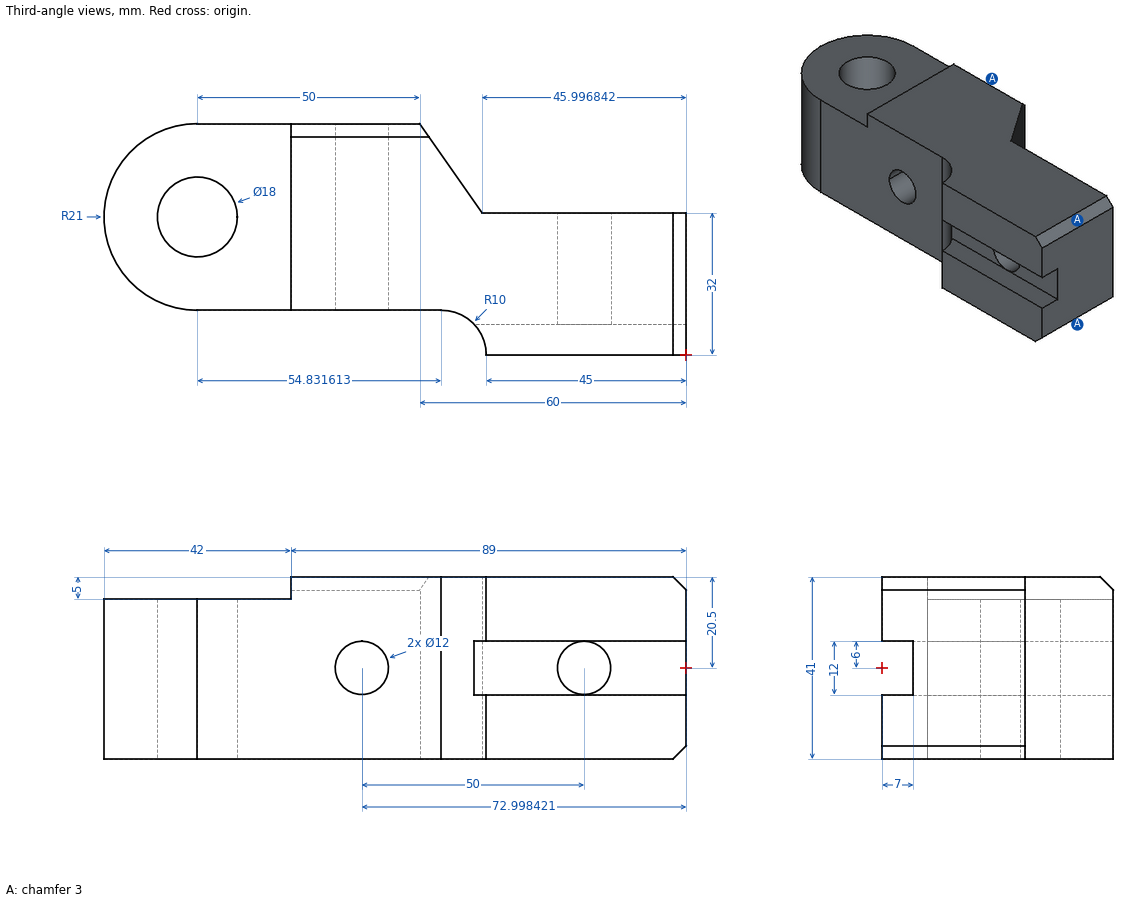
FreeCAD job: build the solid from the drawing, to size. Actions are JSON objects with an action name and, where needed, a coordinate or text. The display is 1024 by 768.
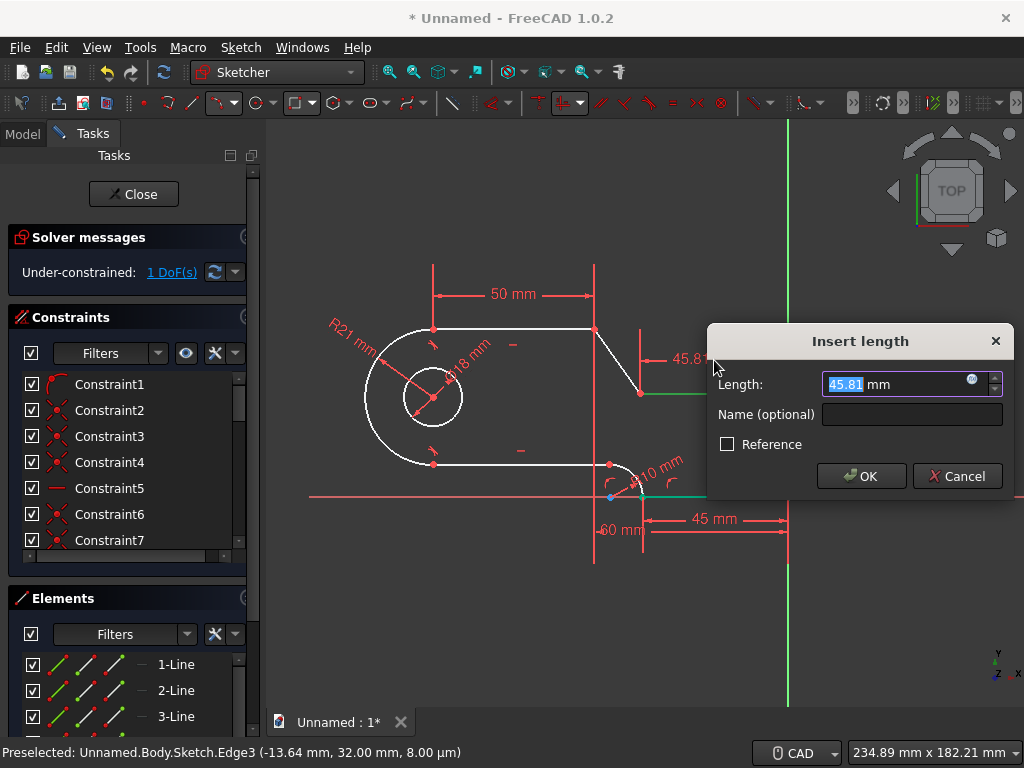
{"action": "type", "text": "45.996842"}
{"action": "key", "text": "Return"}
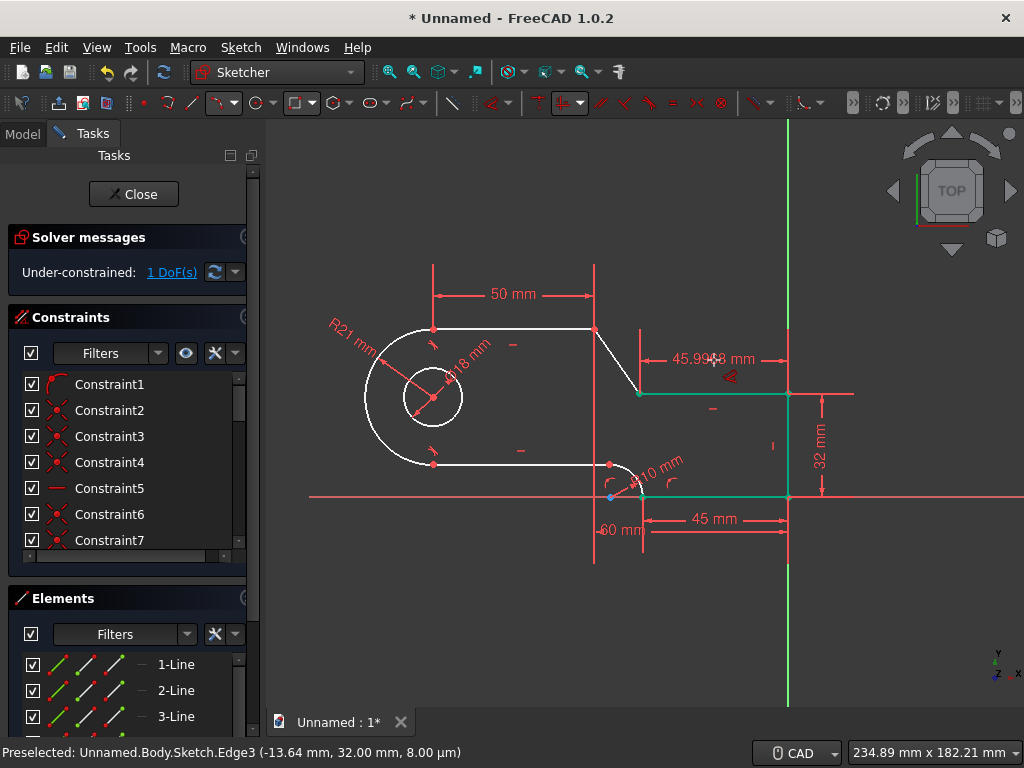
{"action": "left_click", "coordinate": [486, 465]}
{"action": "left_click", "coordinate": [521, 431]}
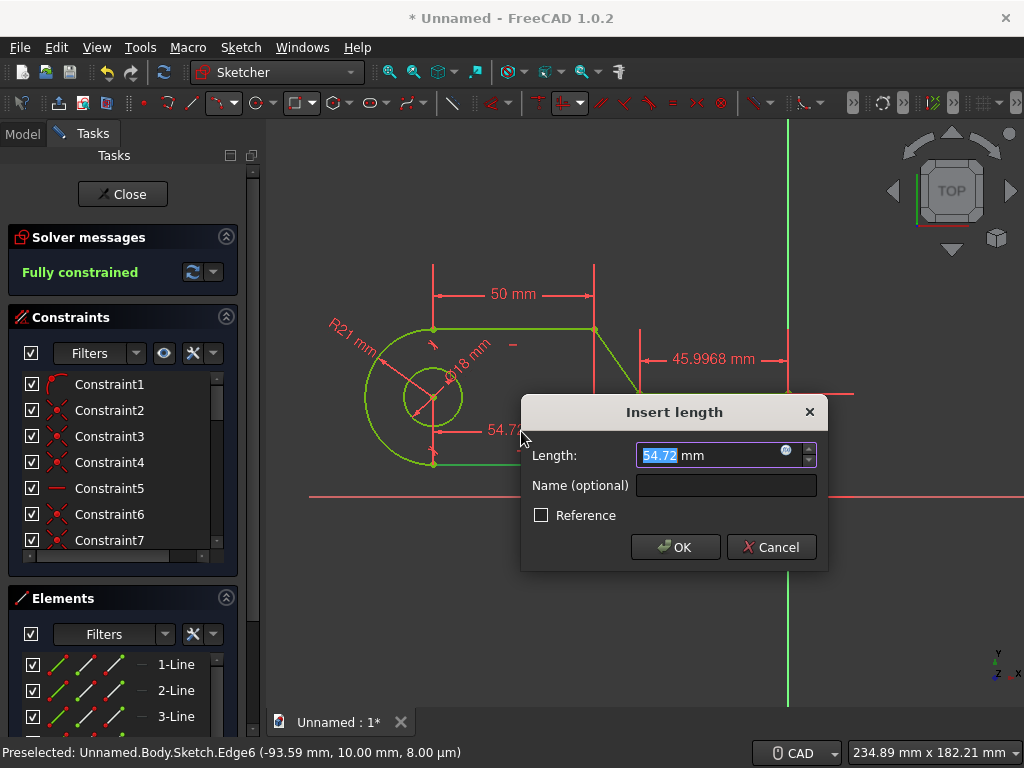
{"action": "type", "text": "54.831613"}
{"action": "key", "text": "Return"}
{"action": "key", "text": "Escape"}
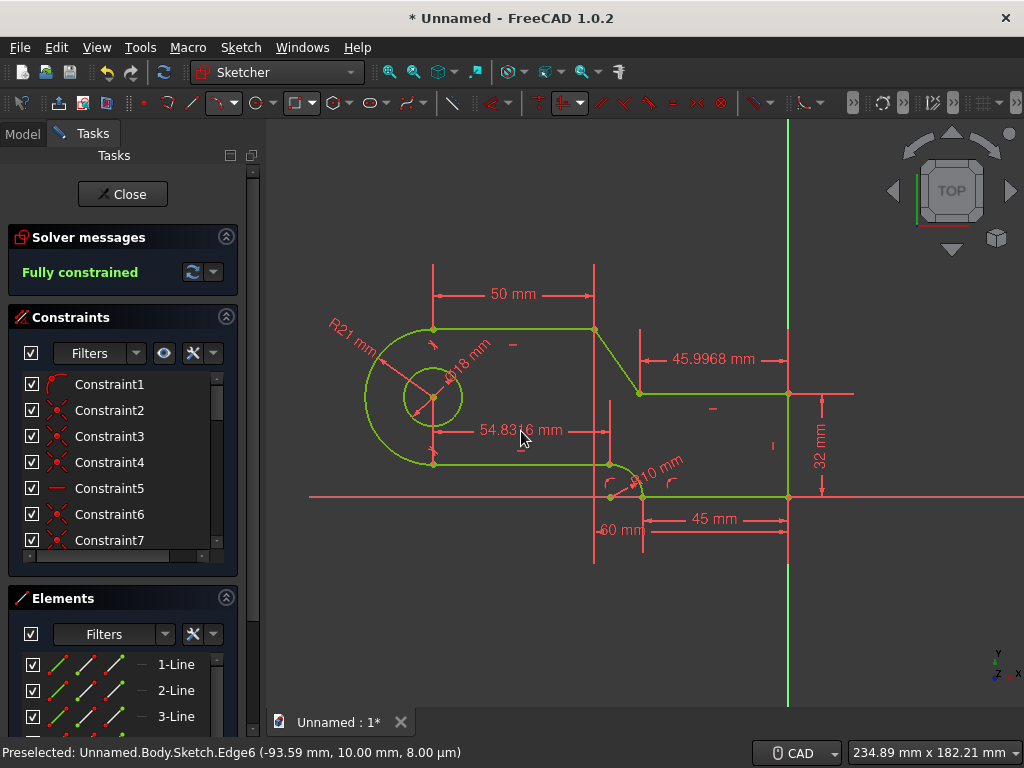
{"action": "left_click", "coordinate": [123, 194]}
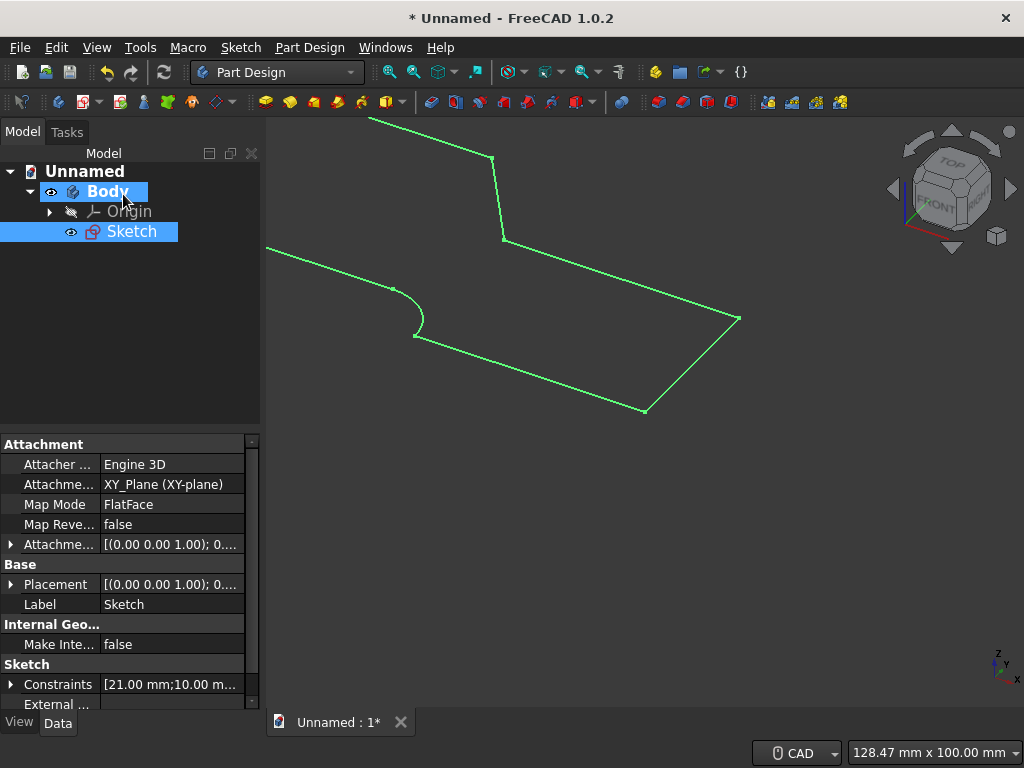
{"action": "left_click", "coordinate": [266, 102]}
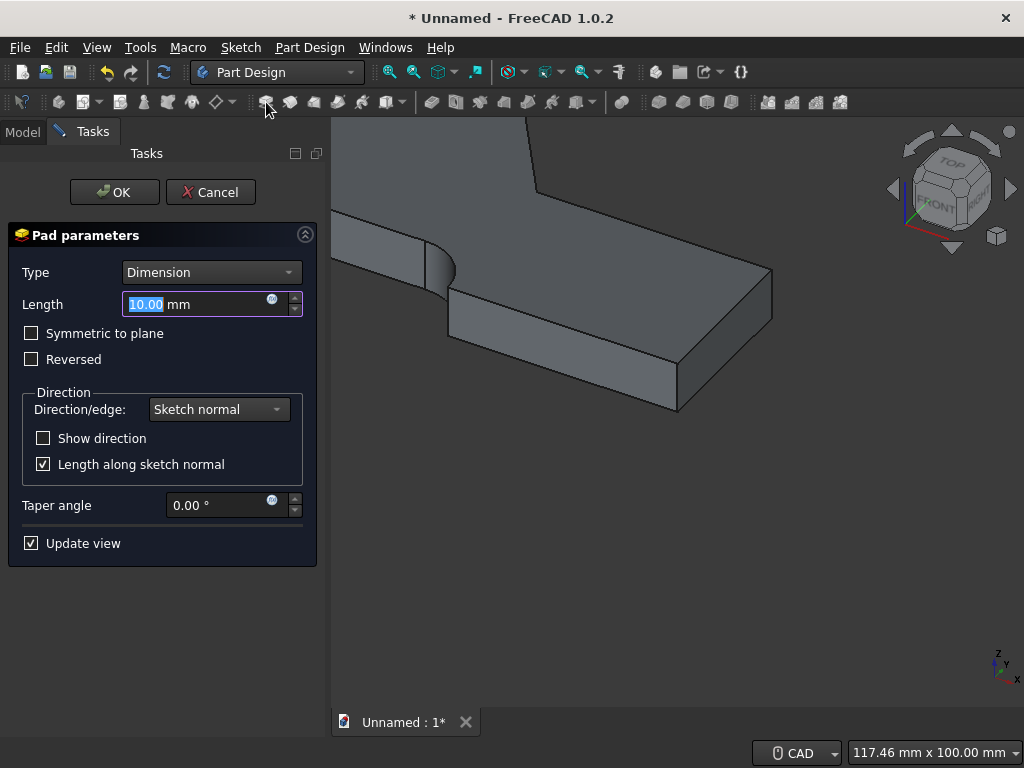
{"action": "type", "text": "41"}
{"action": "key", "text": "Tab"}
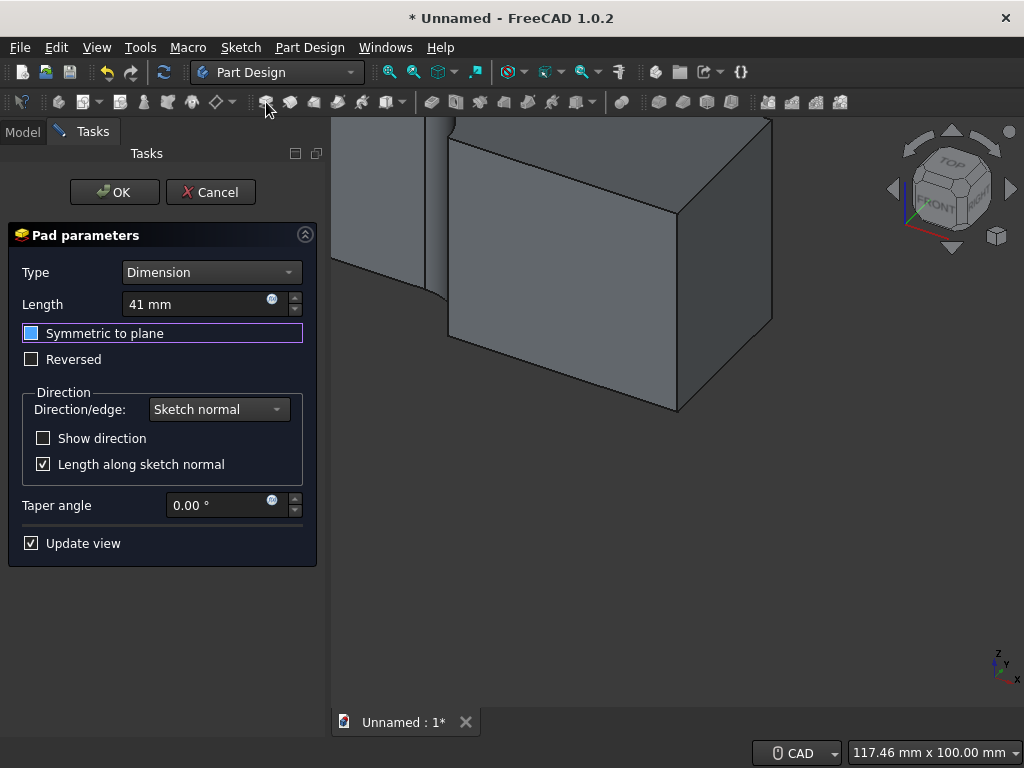
{"action": "left_click", "coordinate": [30, 333]}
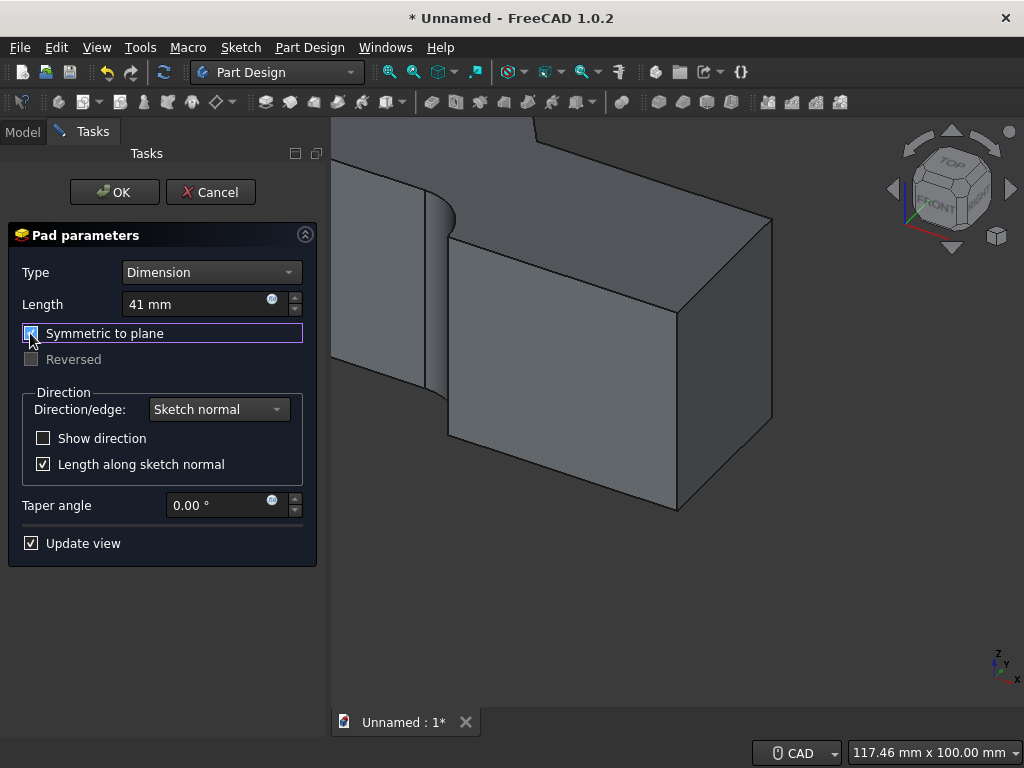
{"action": "left_click", "coordinate": [115, 192]}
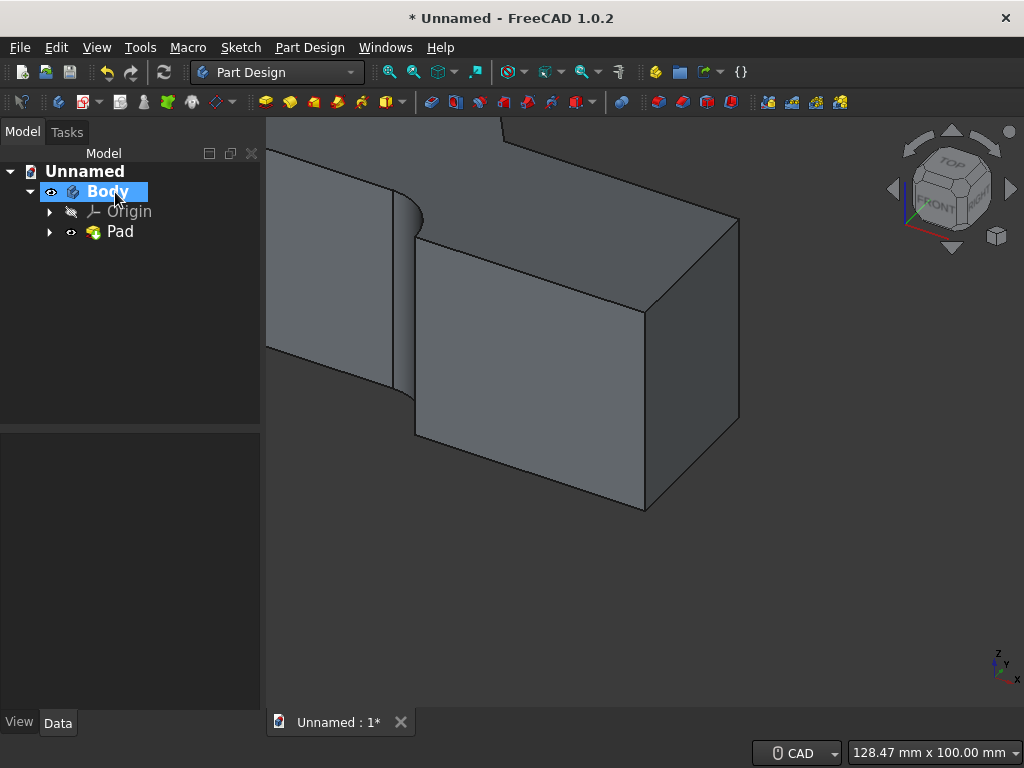
{"action": "left_click", "coordinate": [390, 72]}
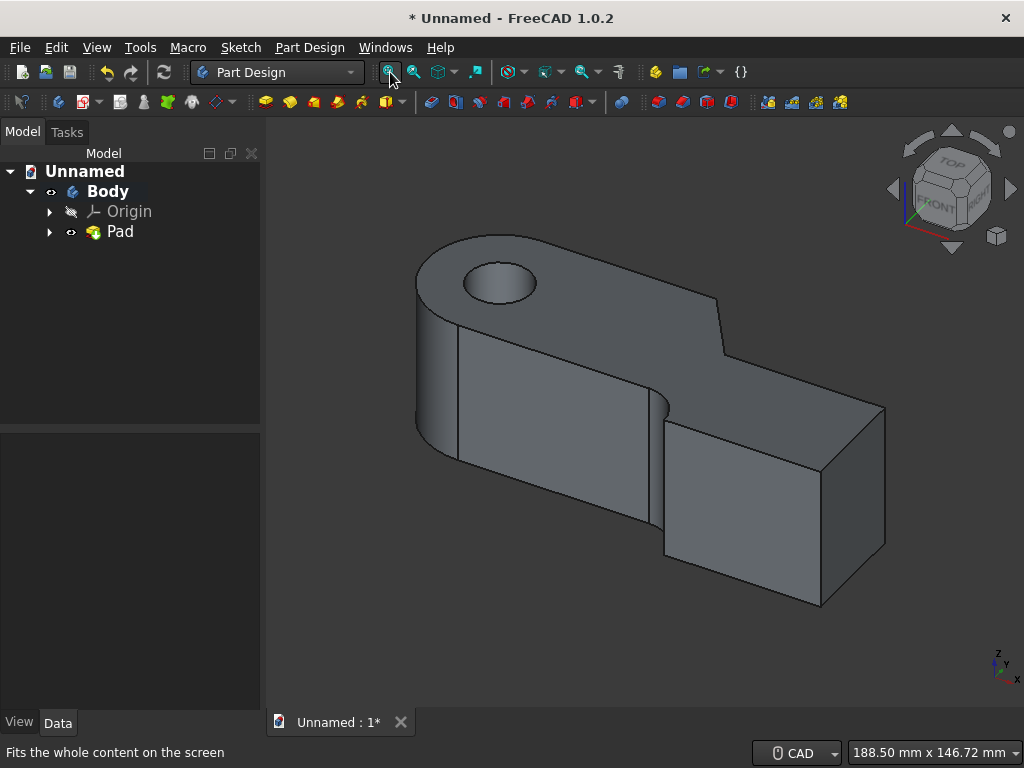
{"action": "key", "text": "4"}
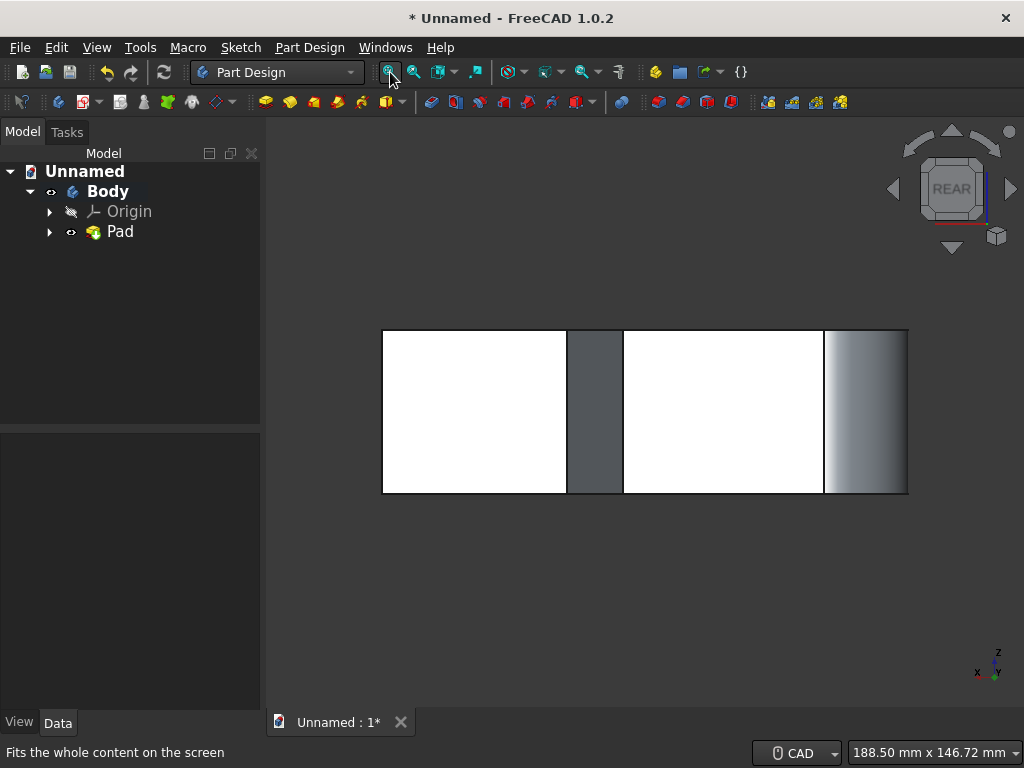
{"action": "left_click", "coordinate": [724, 411]}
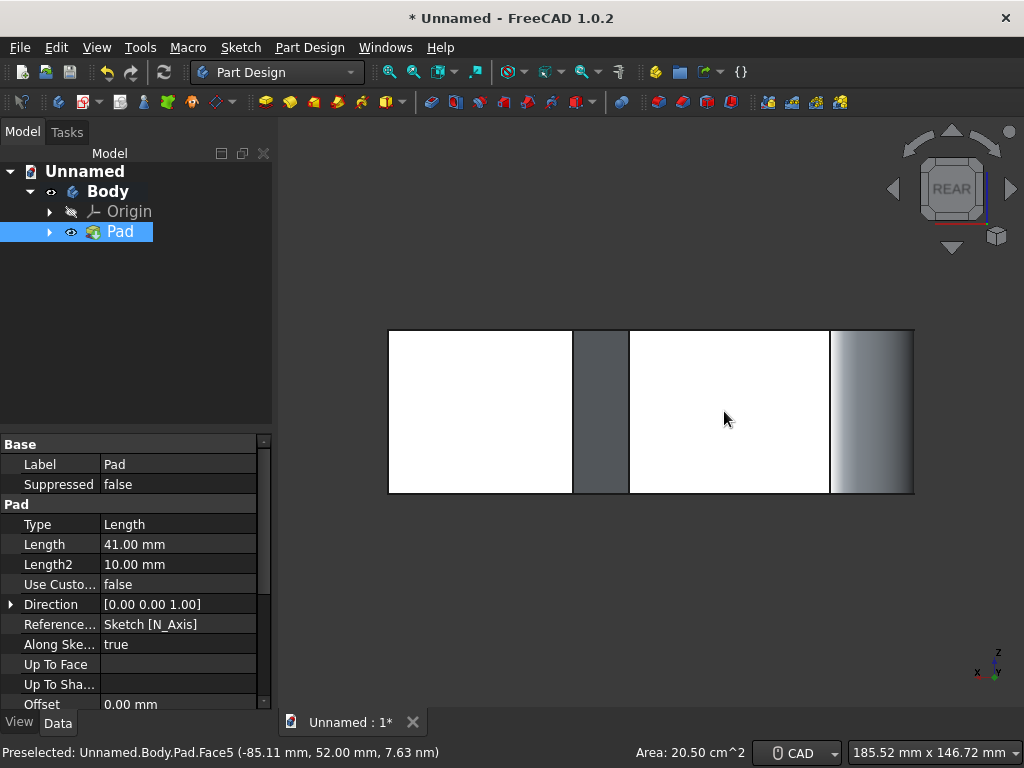
{"action": "left_click", "coordinate": [84, 102]}